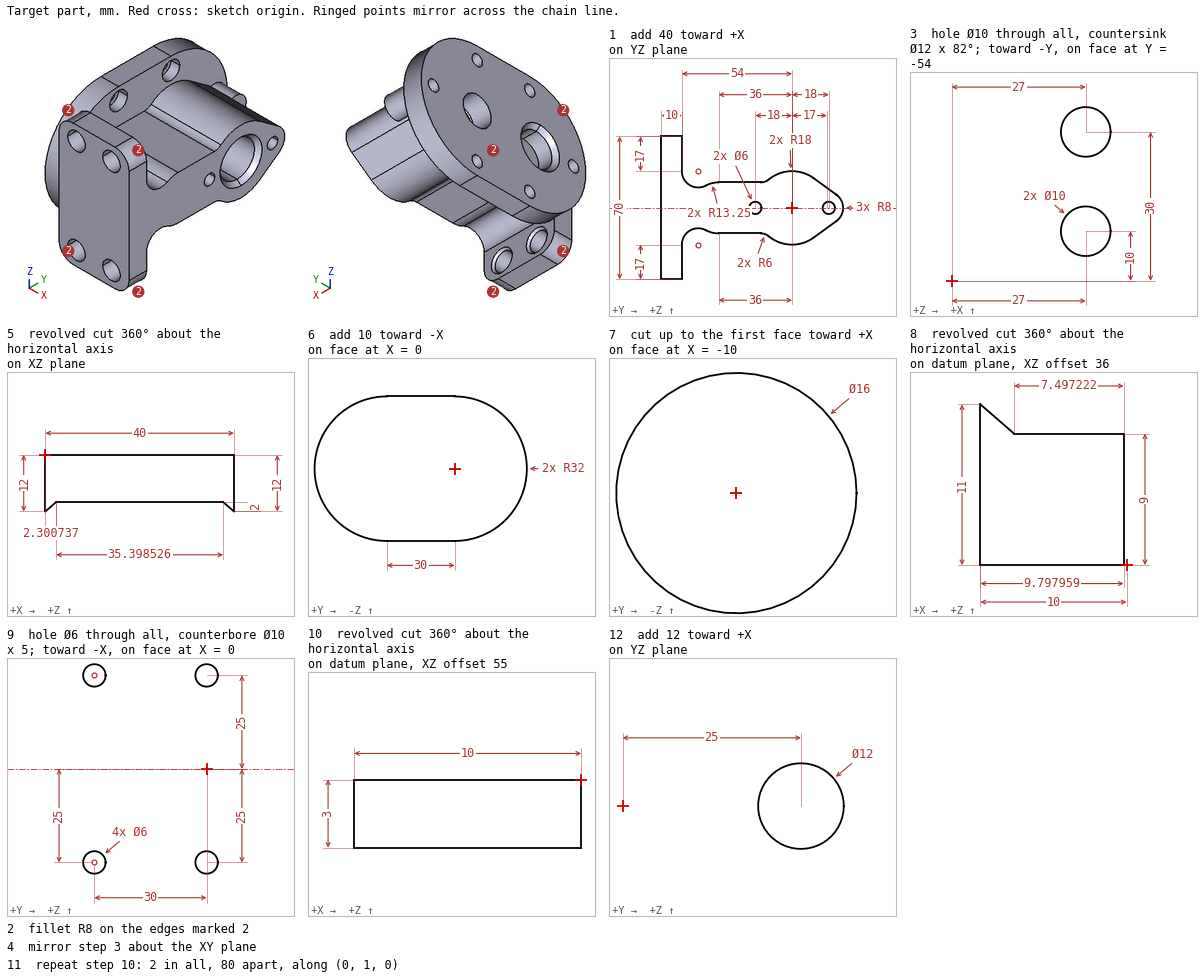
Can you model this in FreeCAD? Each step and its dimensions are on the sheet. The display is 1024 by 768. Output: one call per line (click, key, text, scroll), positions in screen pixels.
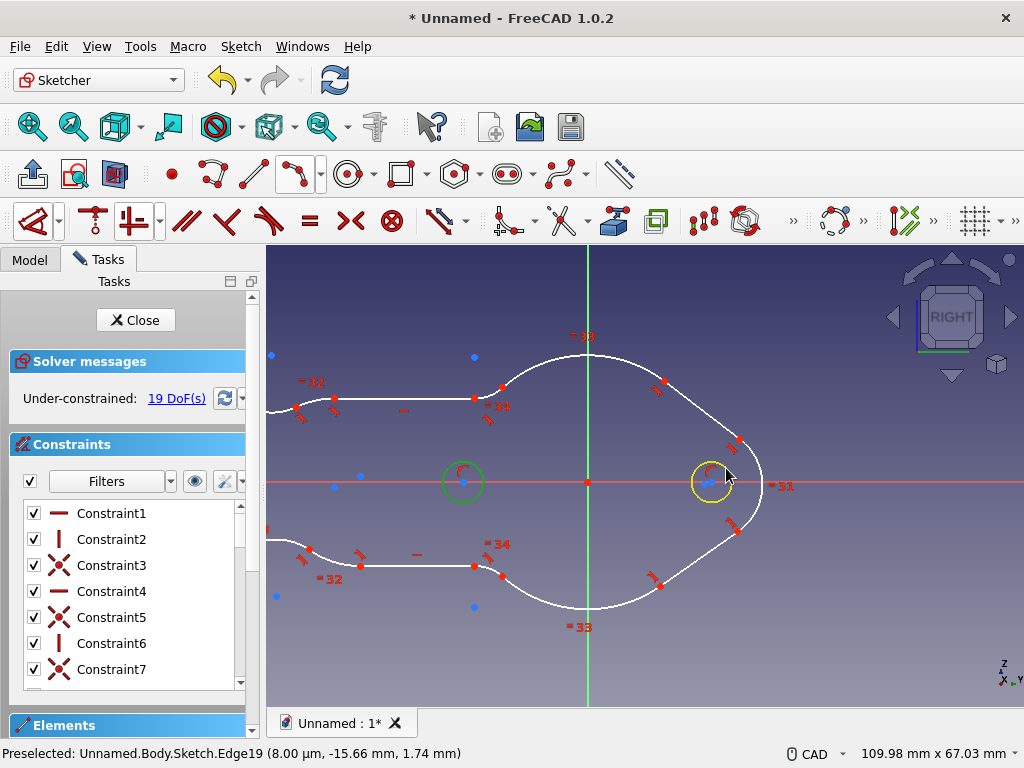
click(726, 468)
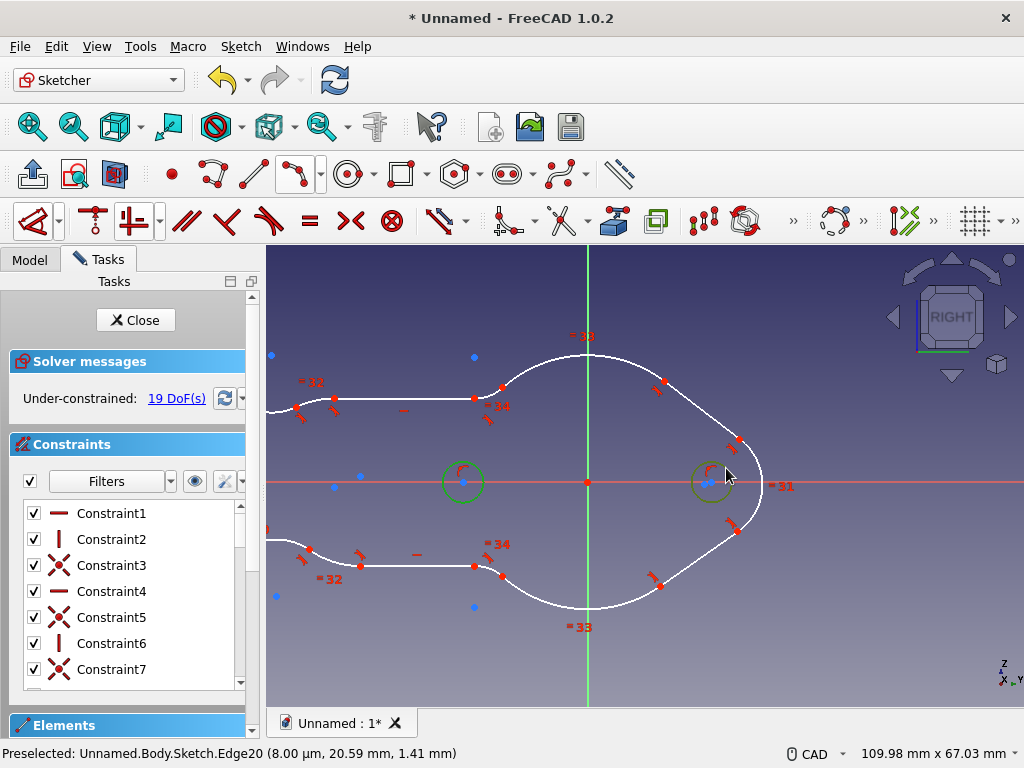
click(310, 222)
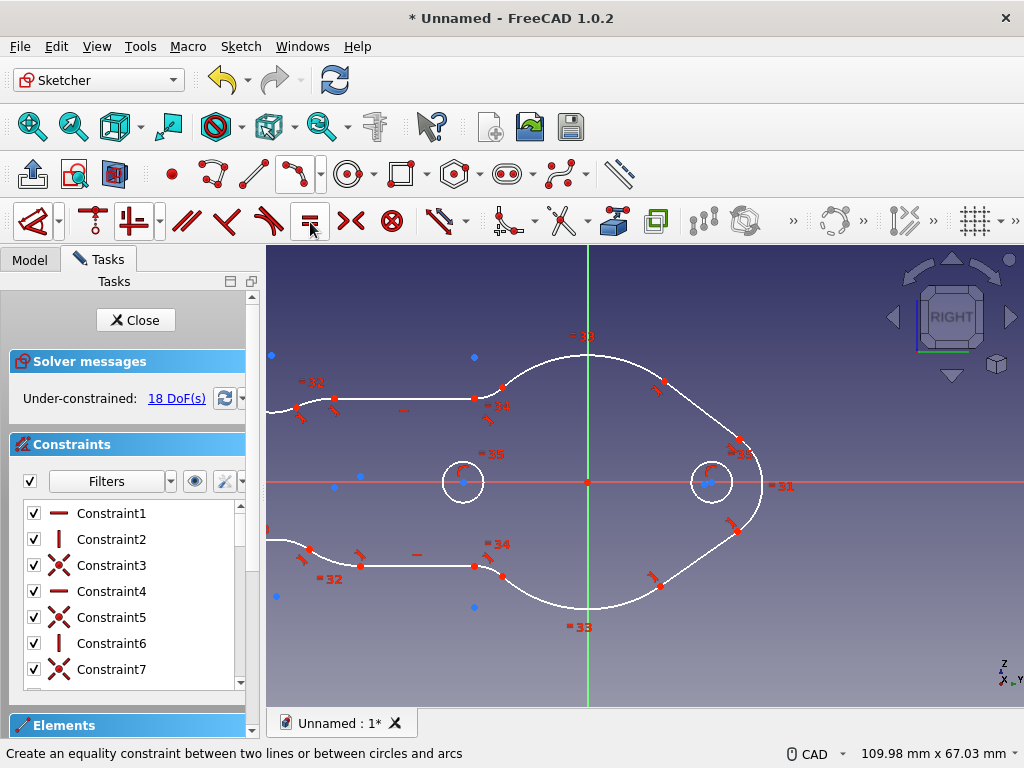
scroll(705, 485, up, 3)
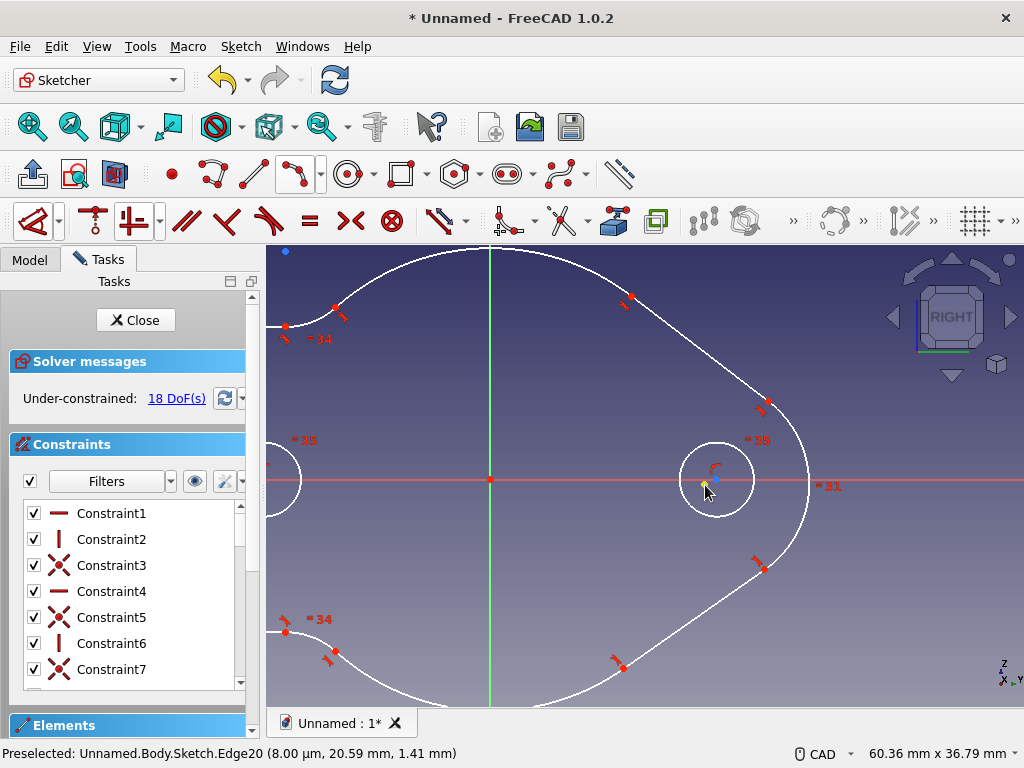
click(705, 484)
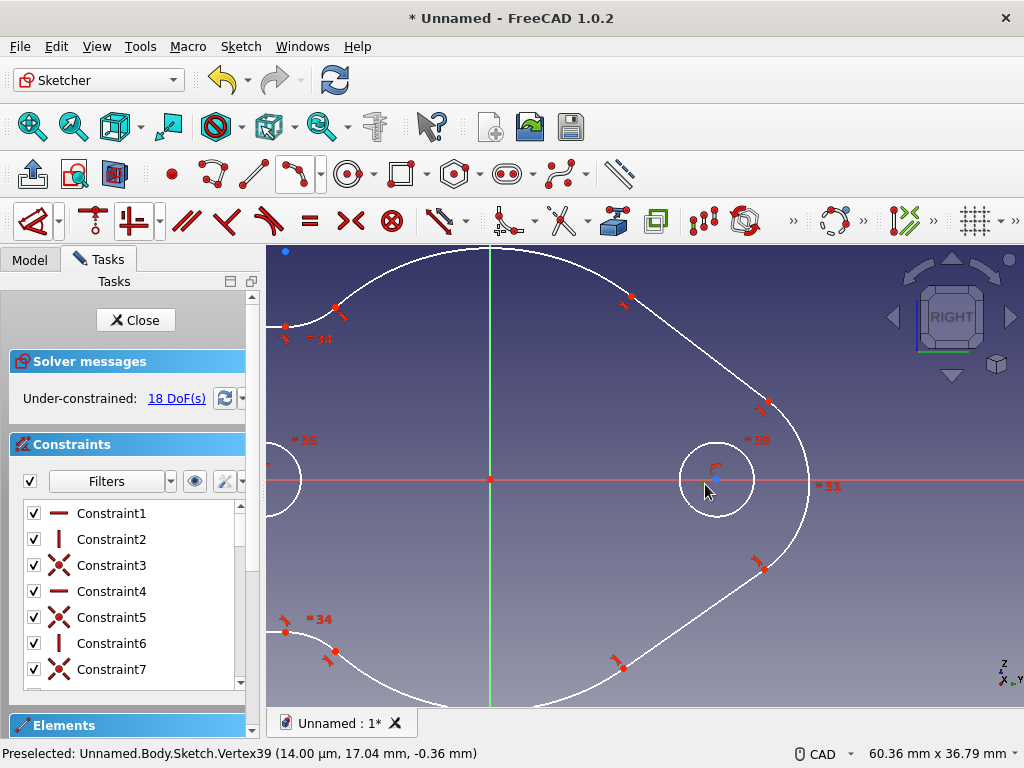
click(334, 480)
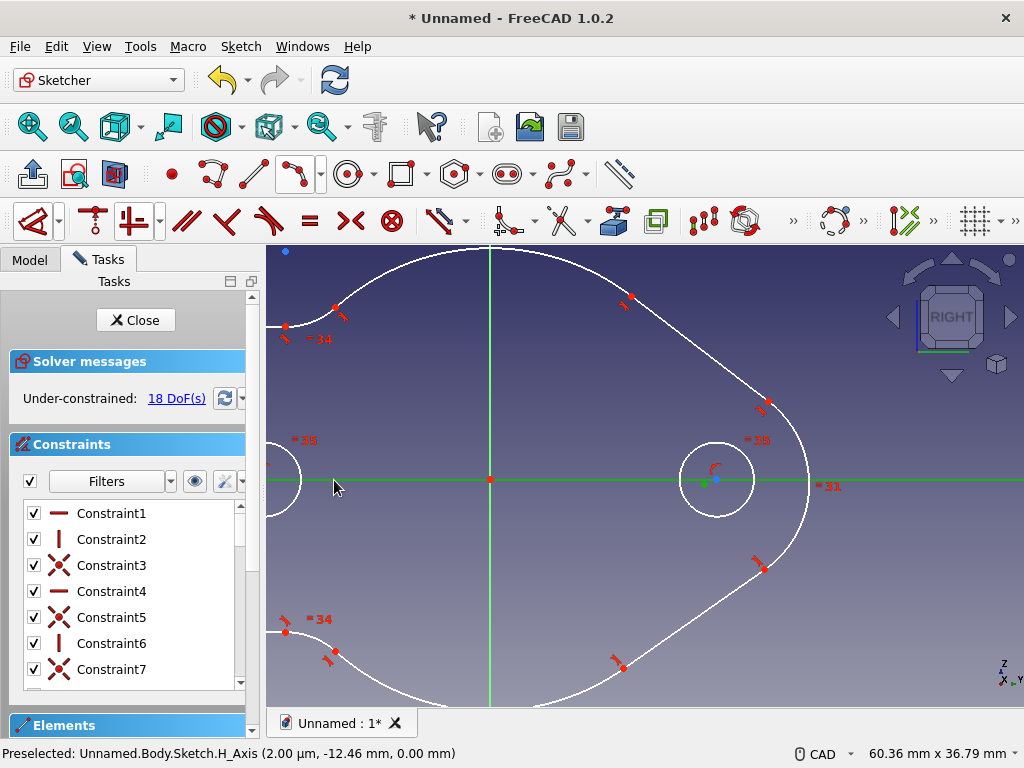
click(93, 222)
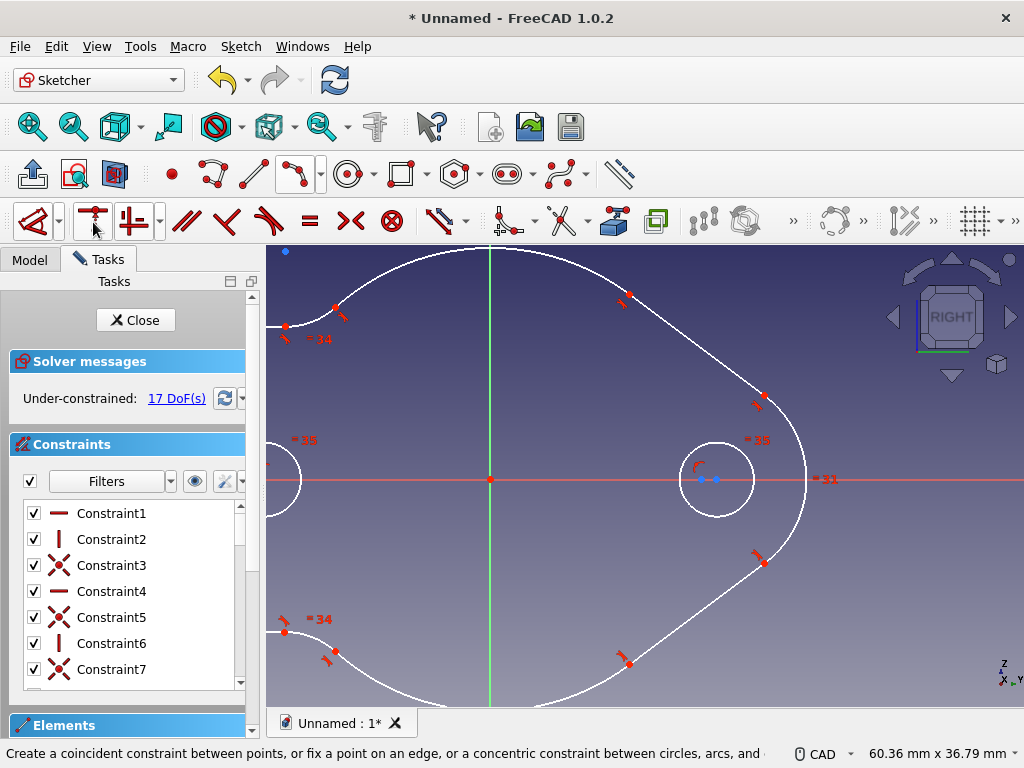
scroll(719, 474, down, 6)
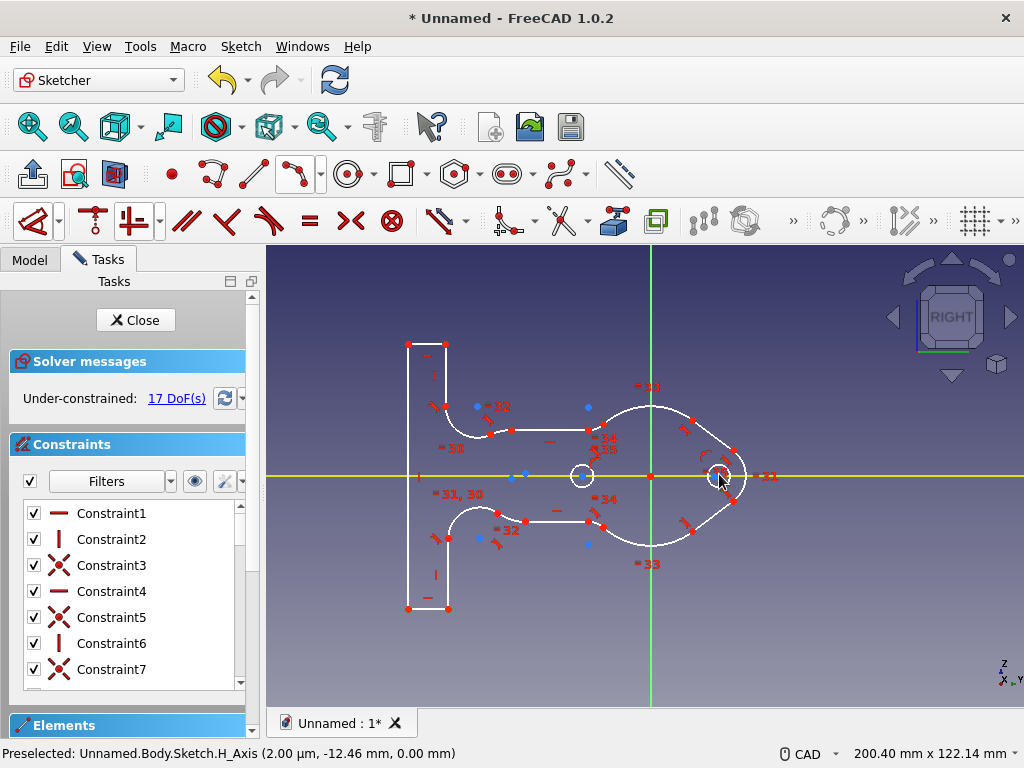
click(477, 406)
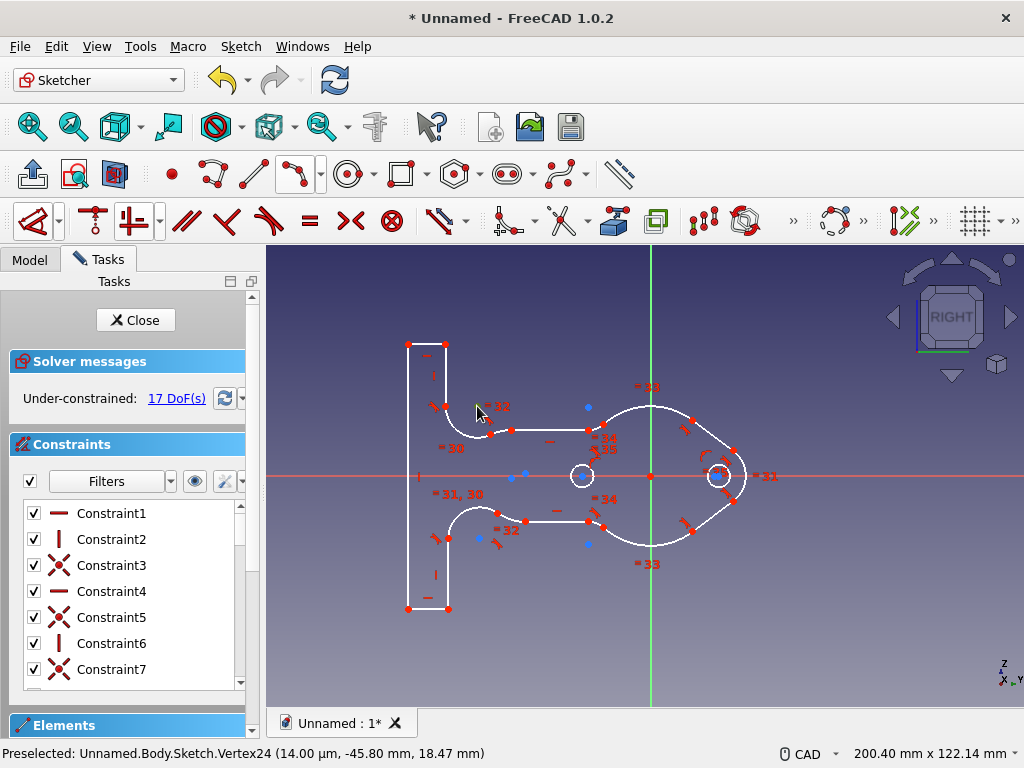
click(480, 539)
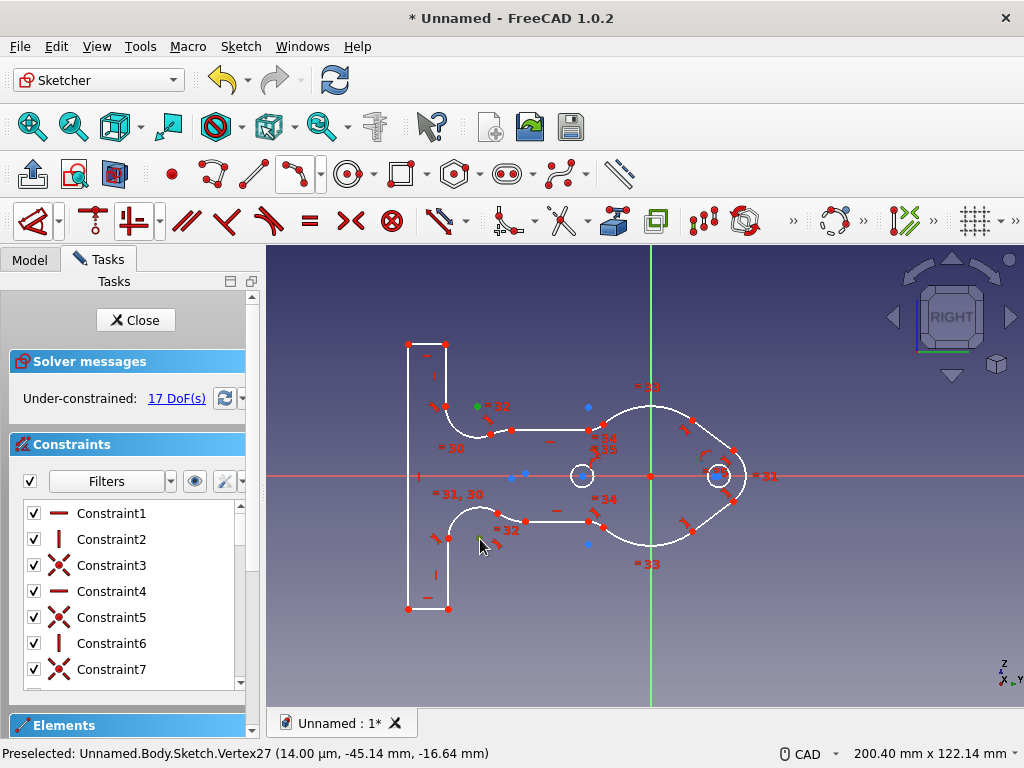
click(334, 476)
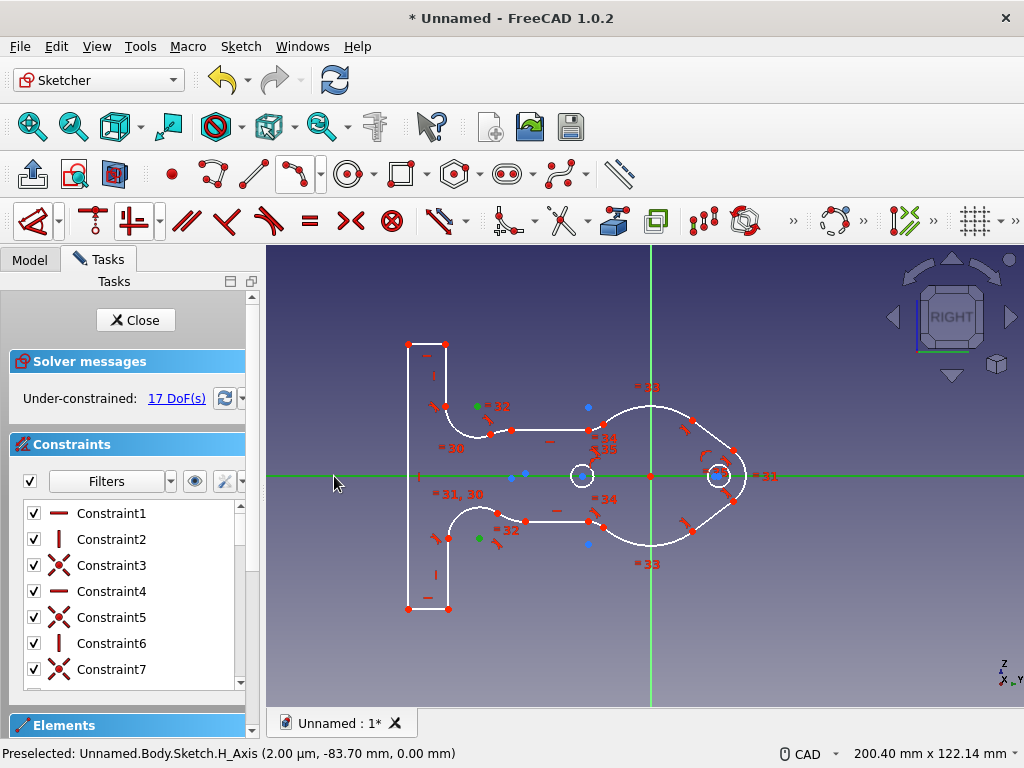
click(351, 222)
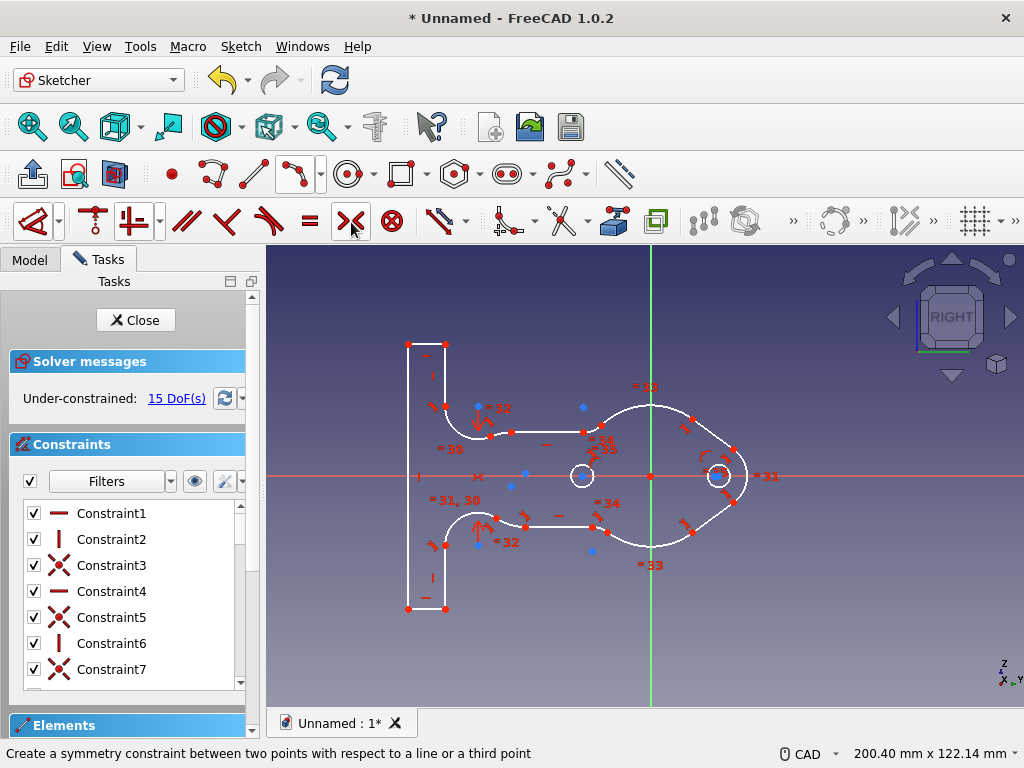
click(32, 222)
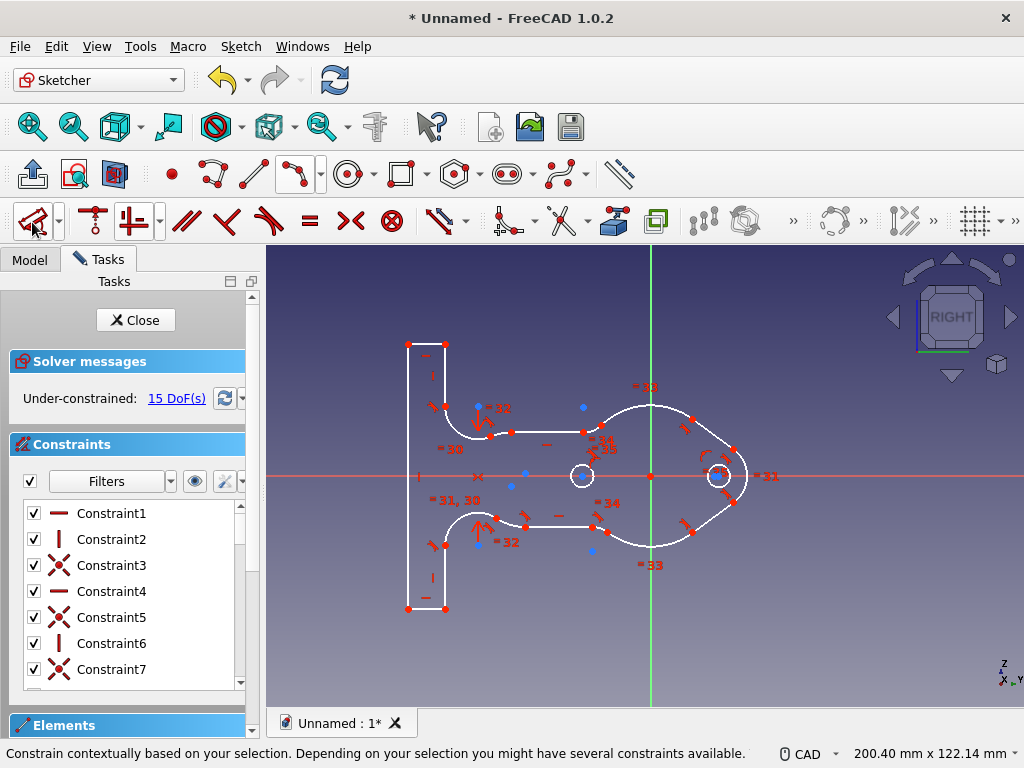
scroll(501, 434, up, 2)